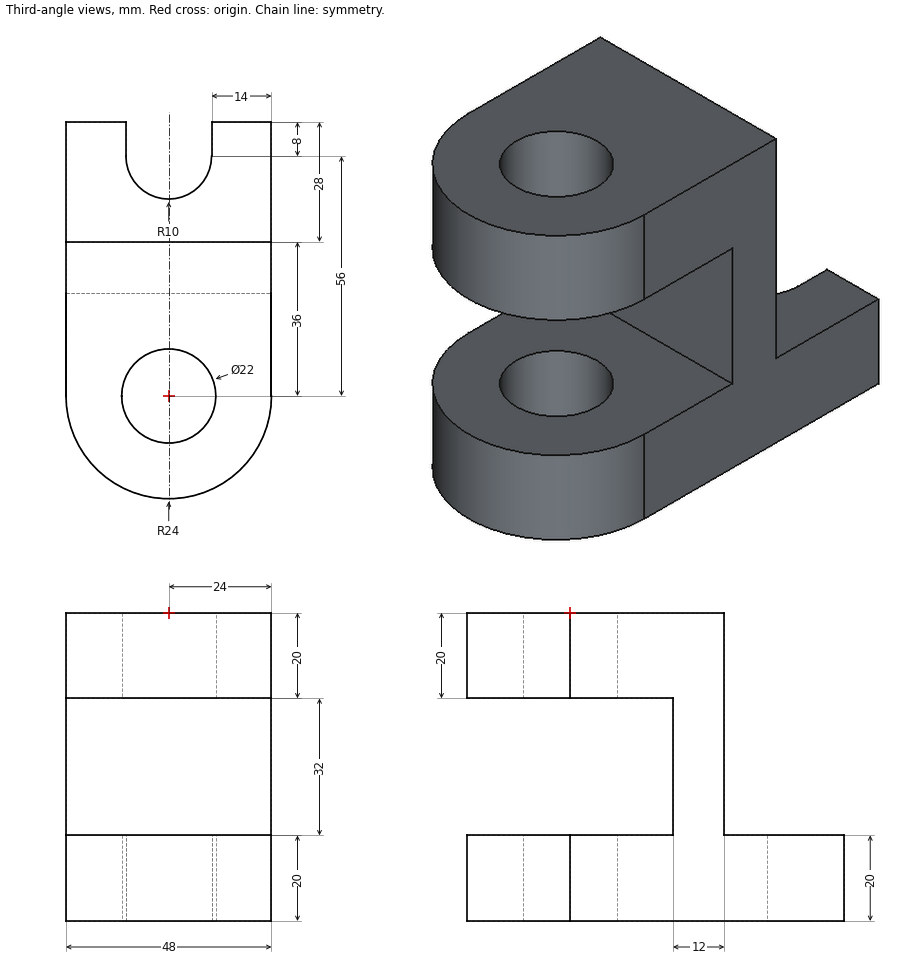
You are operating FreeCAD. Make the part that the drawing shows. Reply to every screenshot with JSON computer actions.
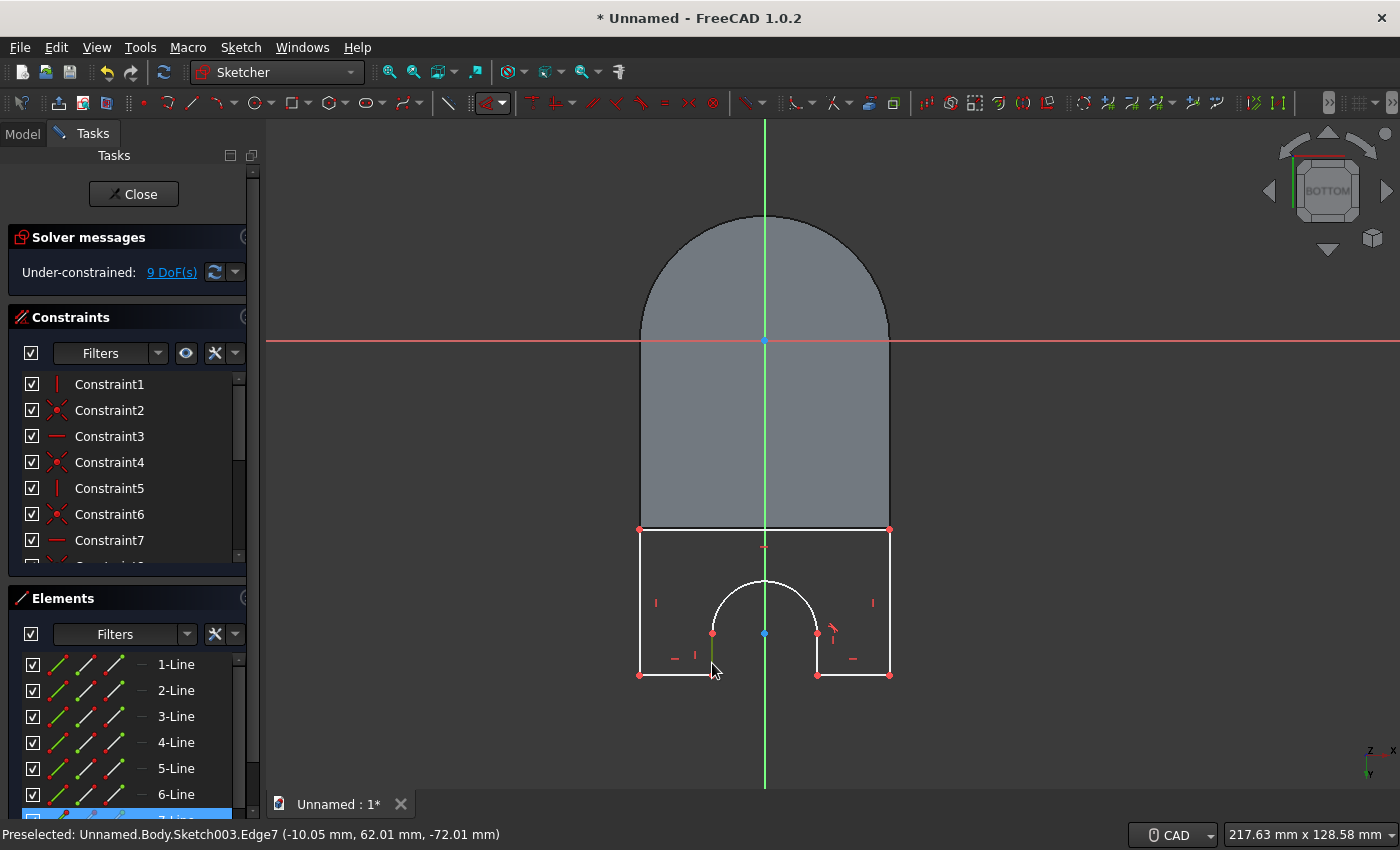
{"action": "left_click", "coordinate": [796, 591]}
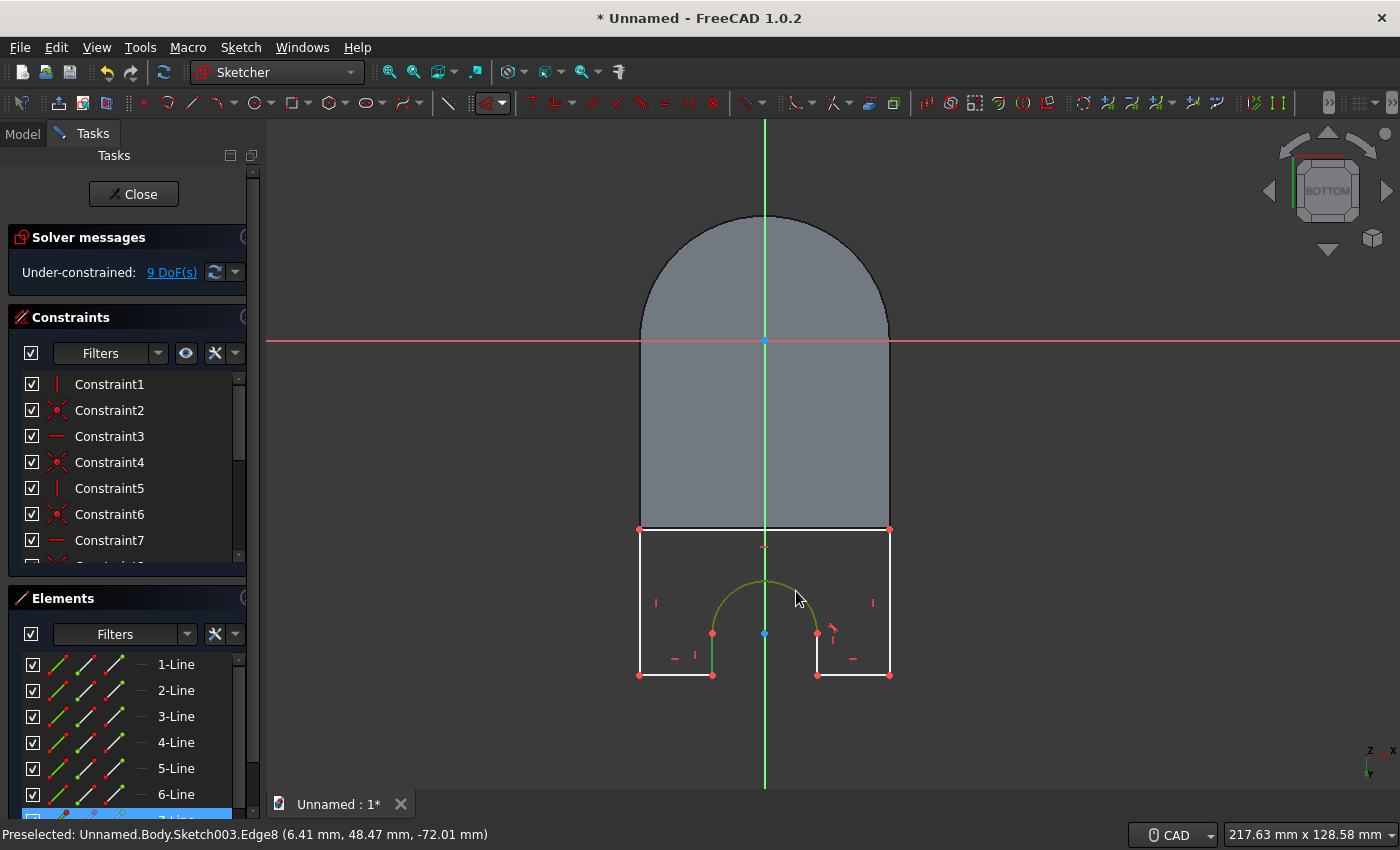
{"action": "left_click", "coordinate": [642, 104]}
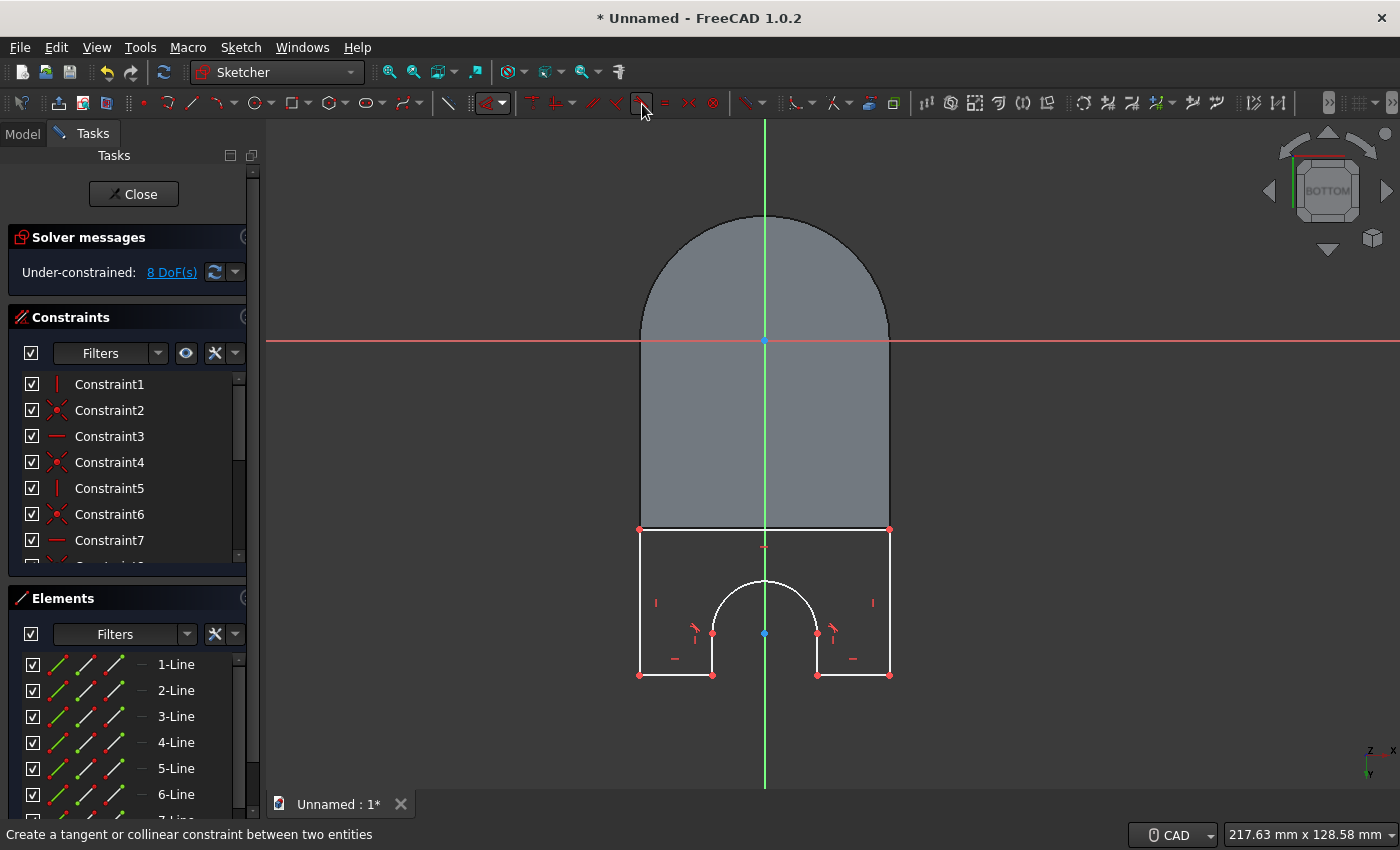
{"action": "left_click", "coordinate": [765, 634]}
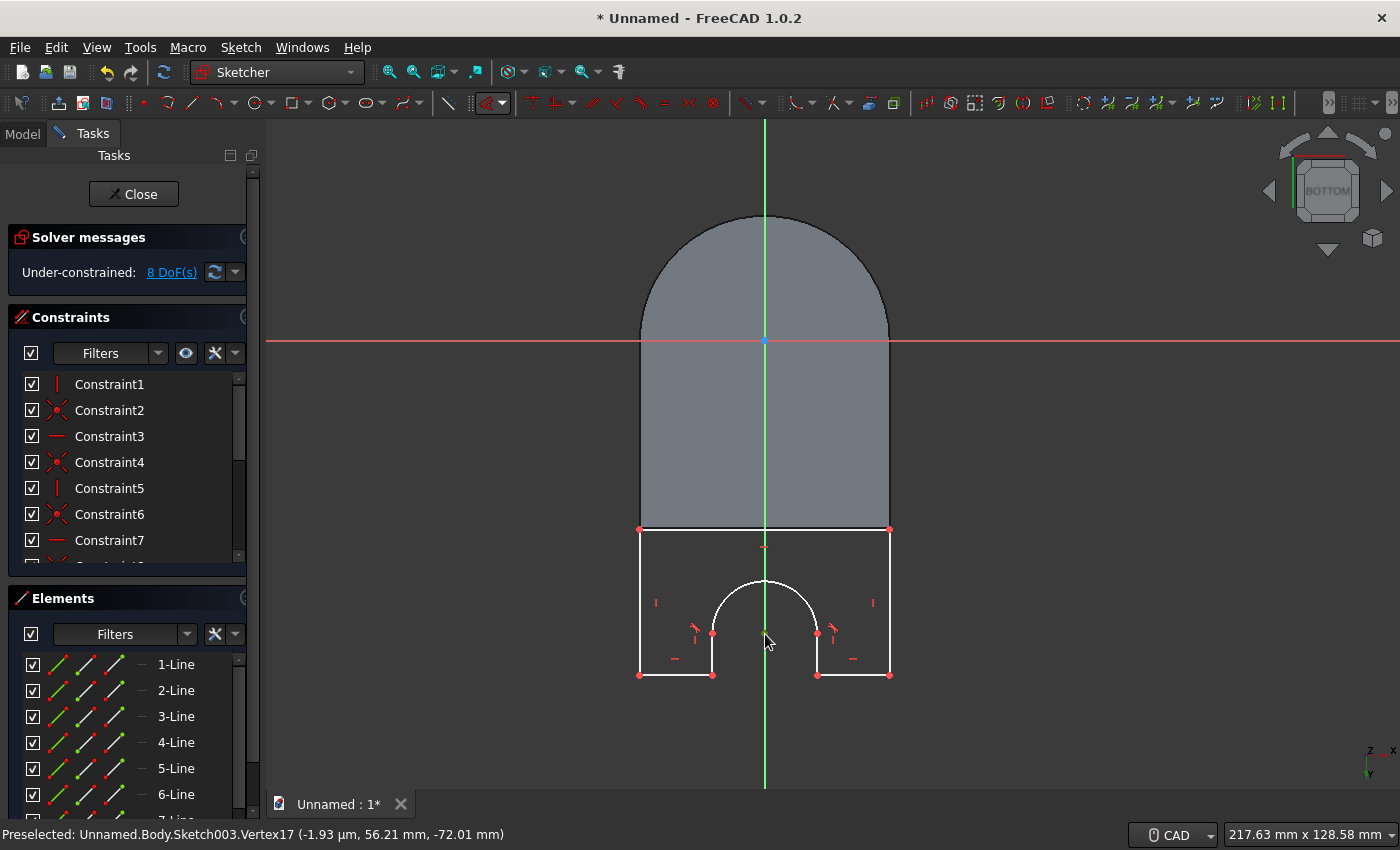
{"action": "left_click", "coordinate": [765, 717]}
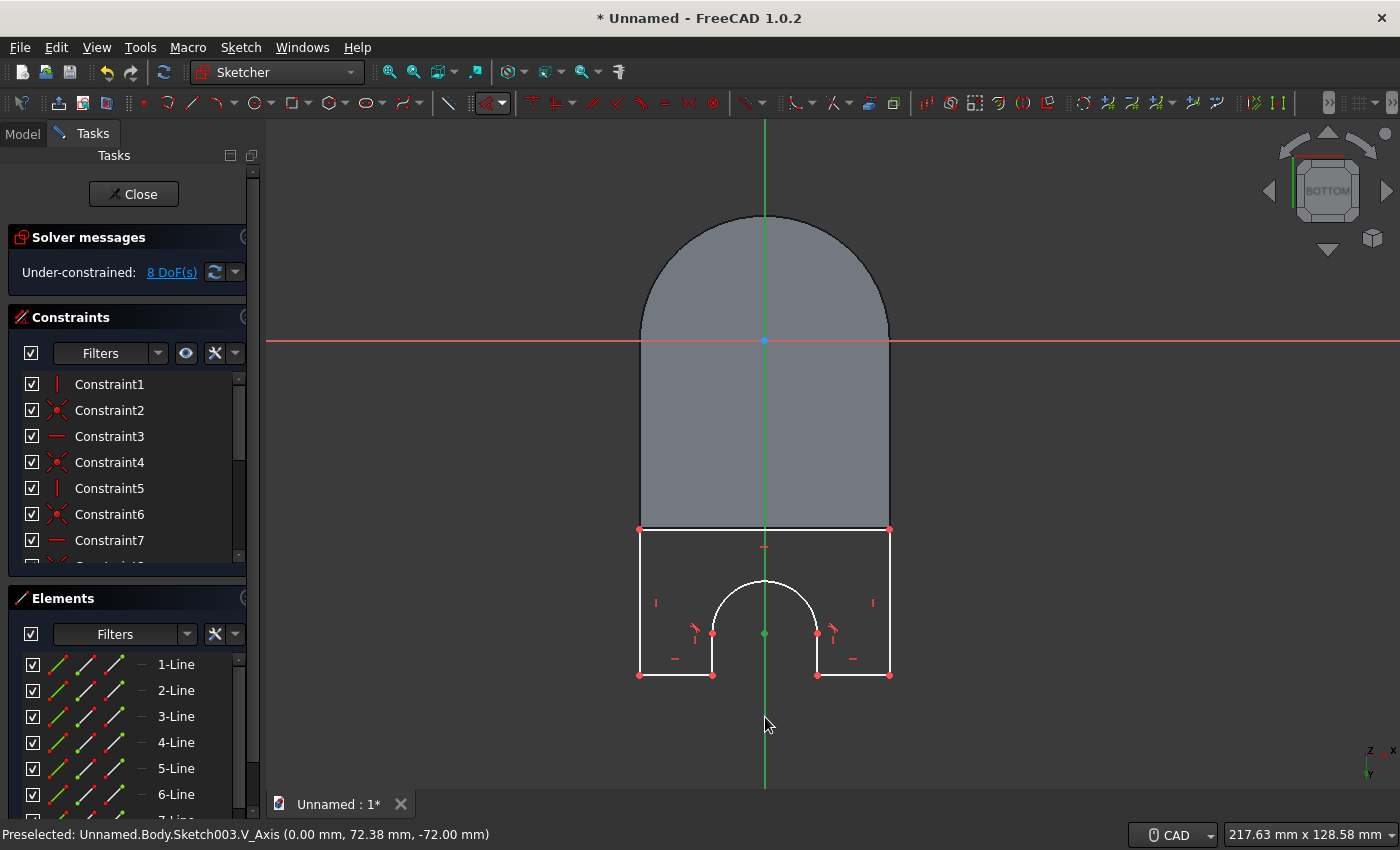
{"action": "left_click", "coordinate": [532, 104]}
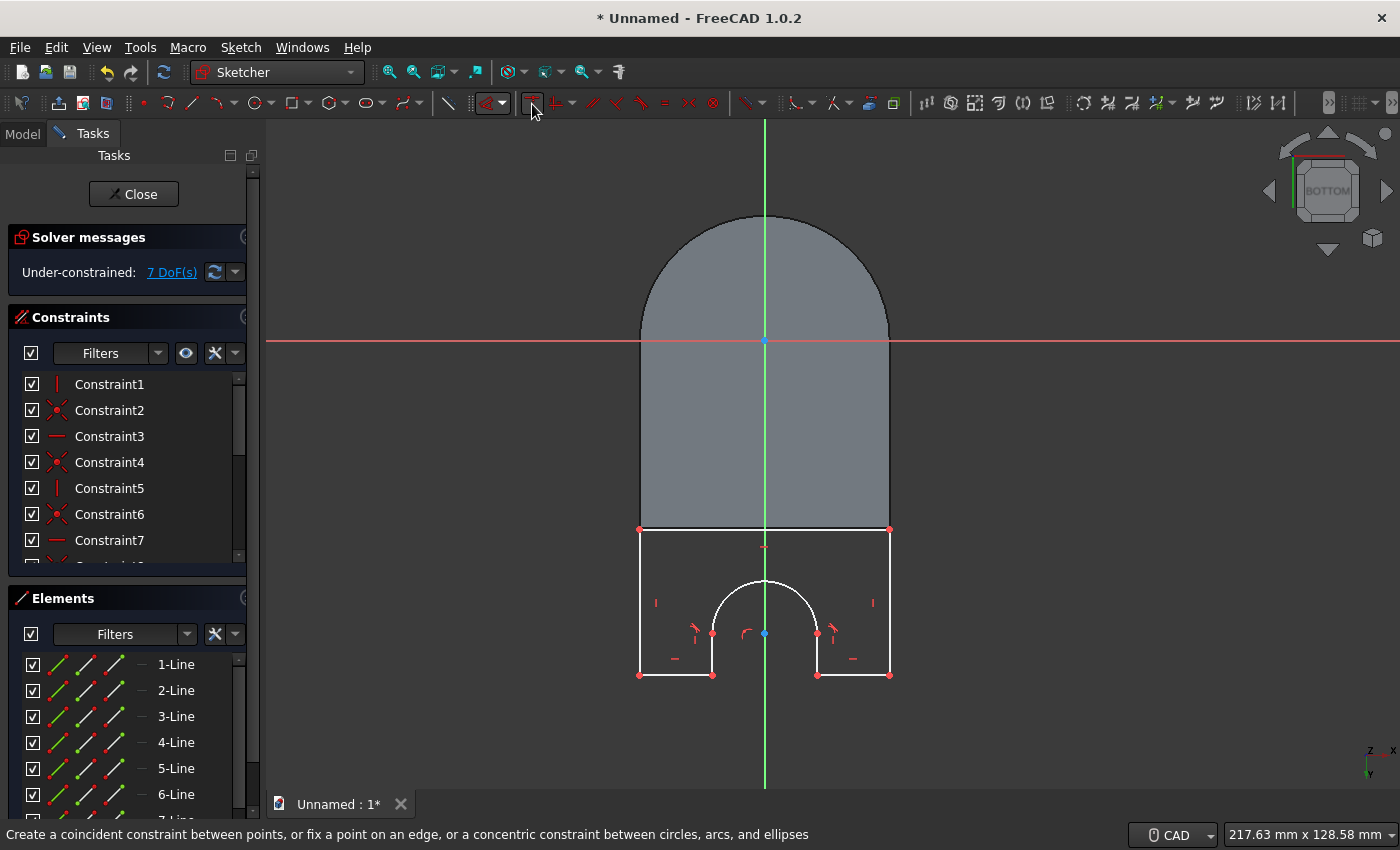
{"action": "left_click", "coordinate": [890, 675]}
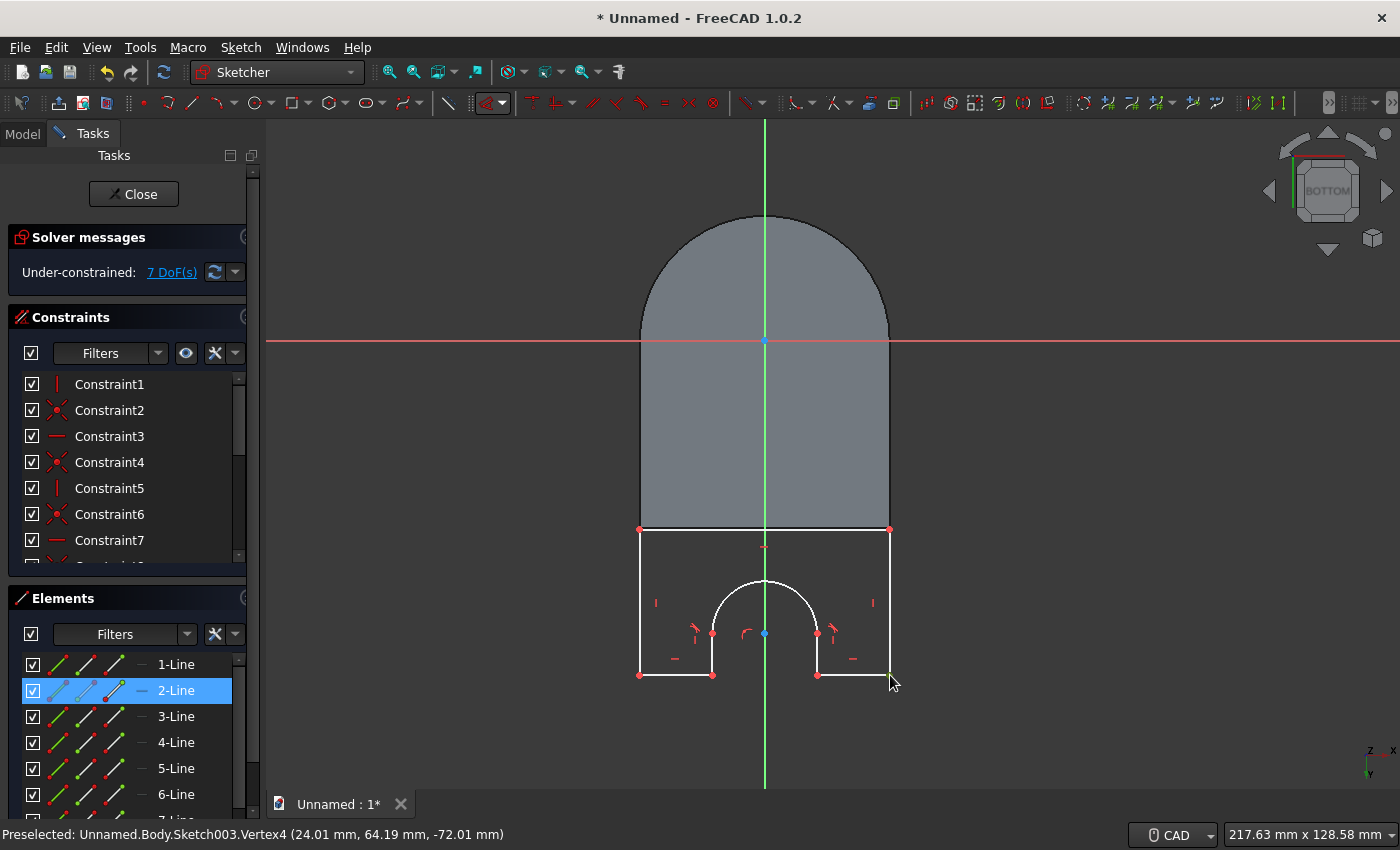
{"action": "left_click", "coordinate": [640, 675]}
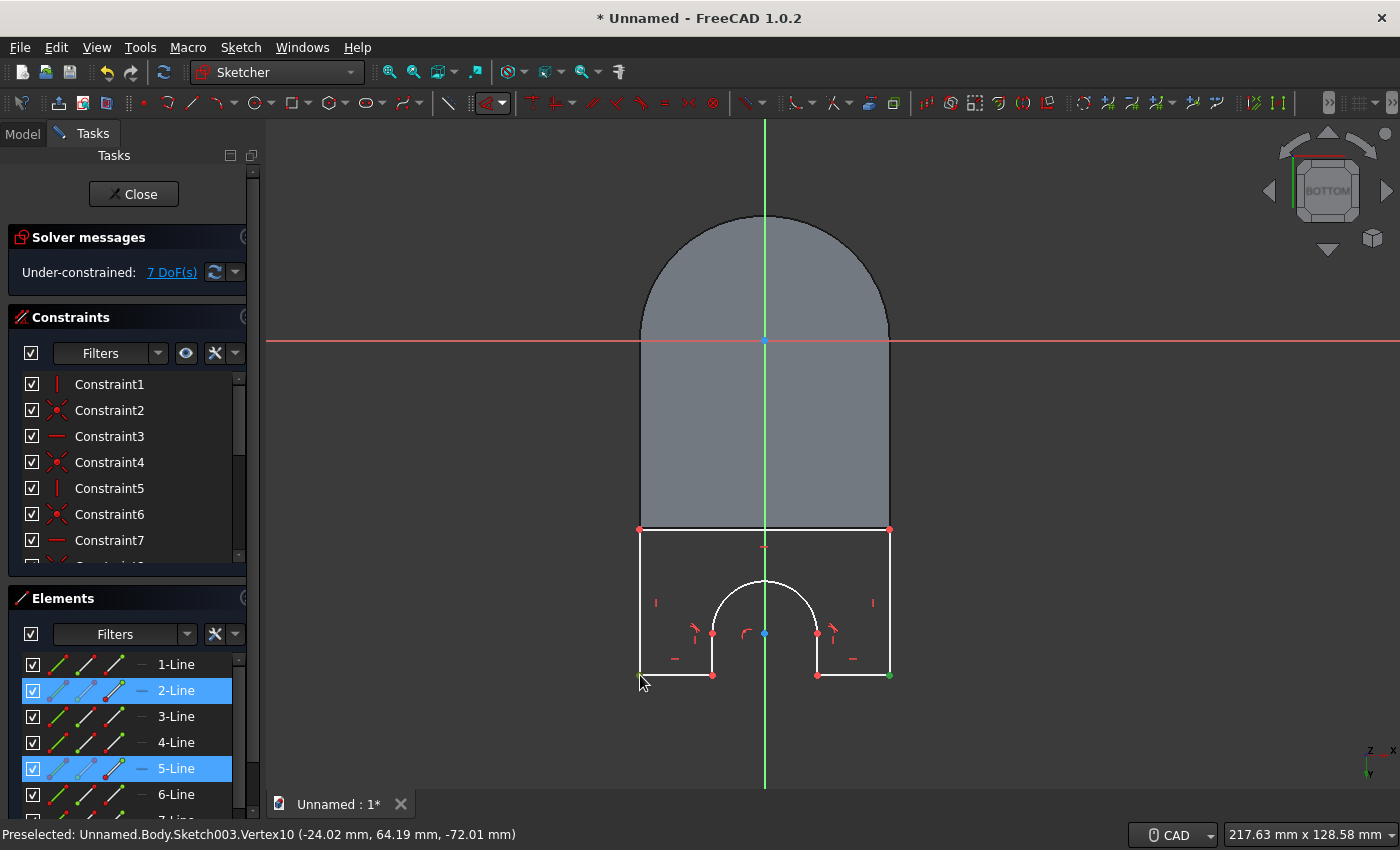
{"action": "left_click", "coordinate": [765, 717]}